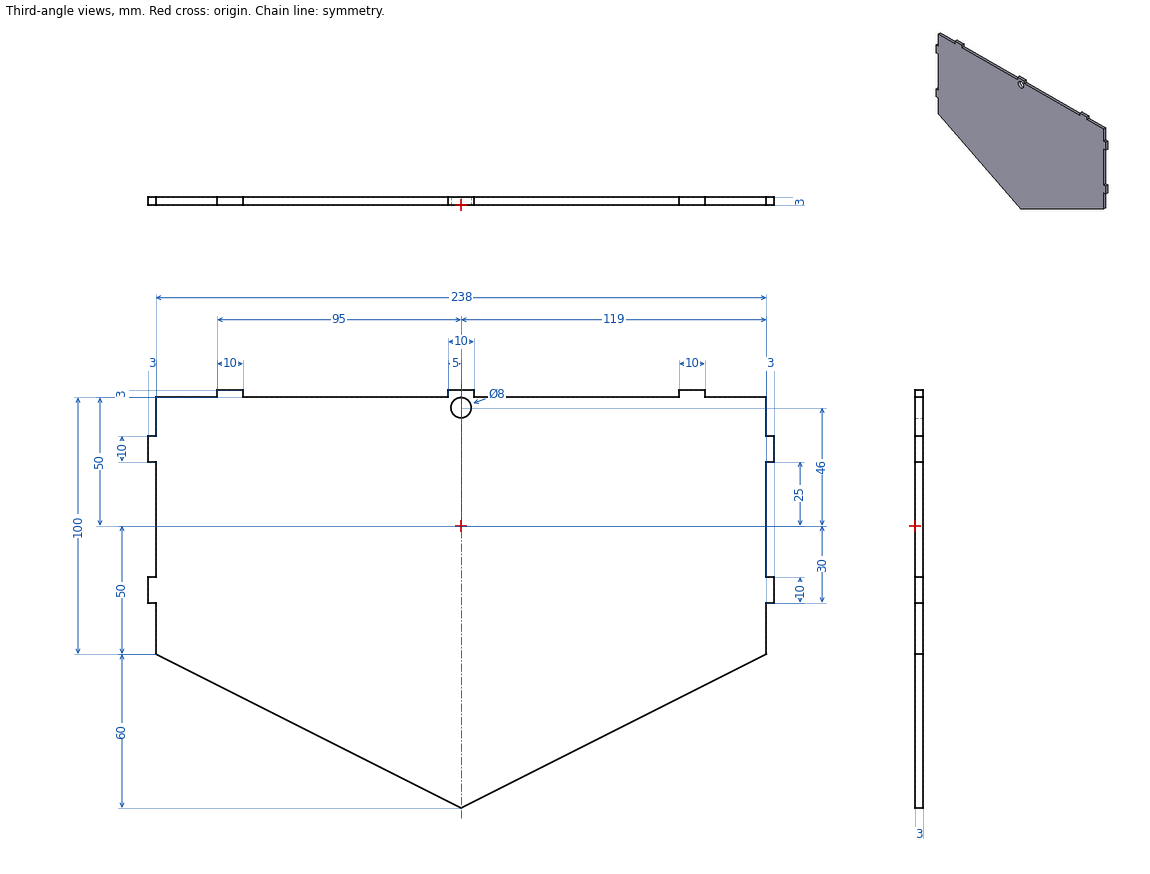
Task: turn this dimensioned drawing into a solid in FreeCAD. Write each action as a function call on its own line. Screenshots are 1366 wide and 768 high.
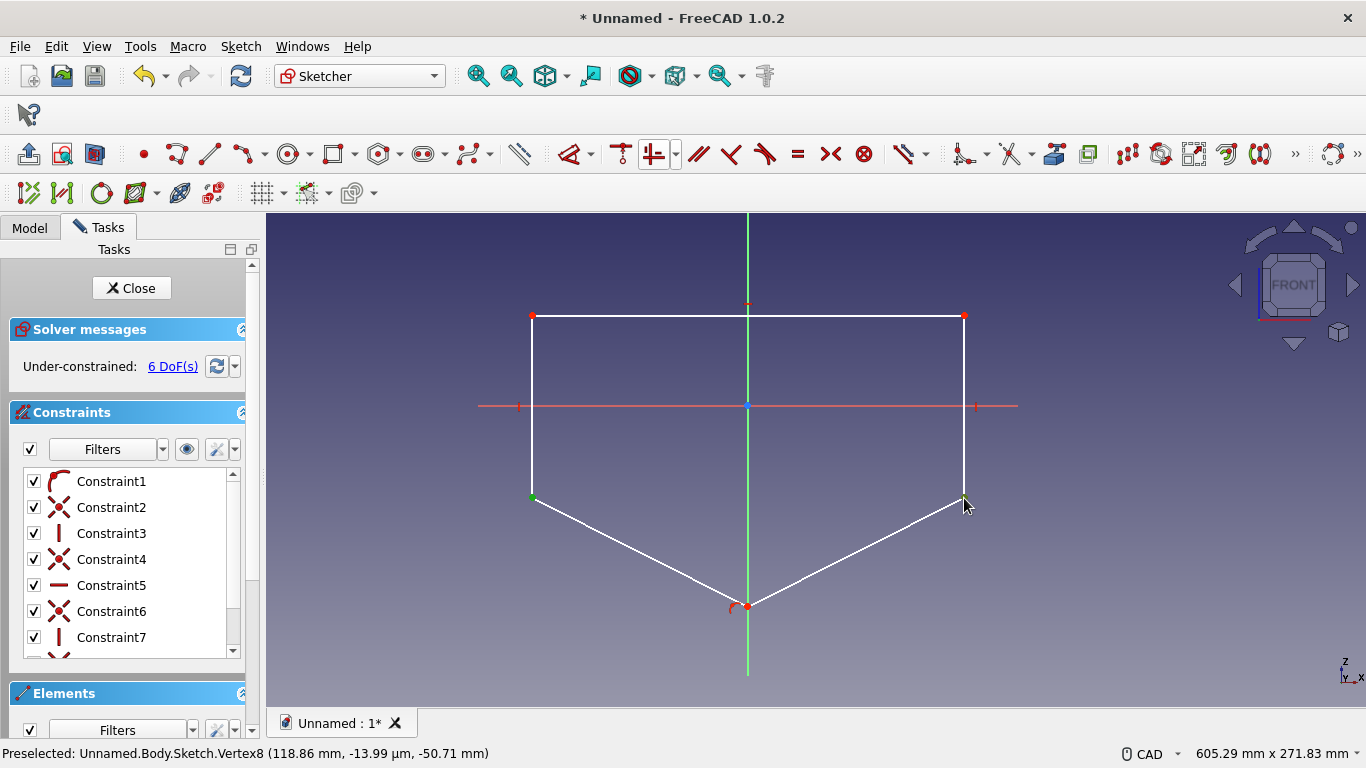
click(748, 648)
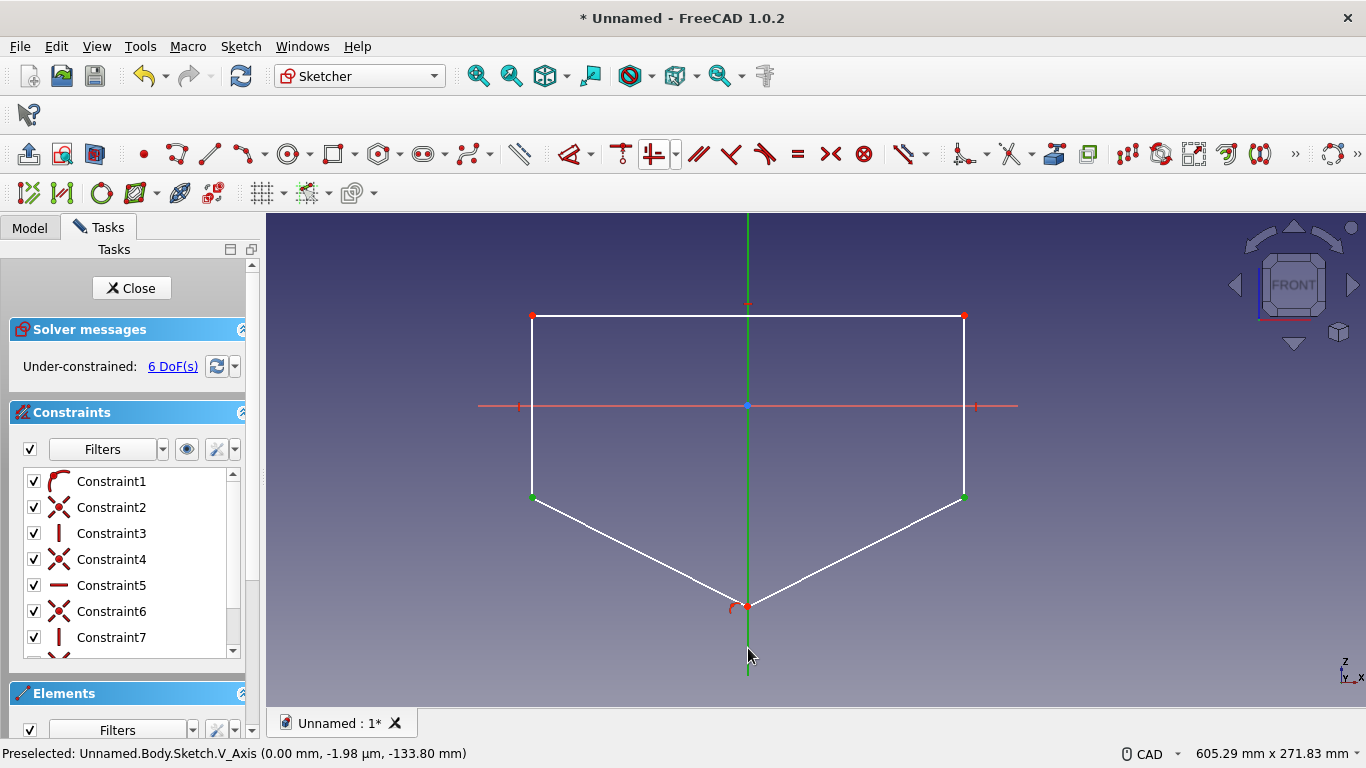
click(831, 154)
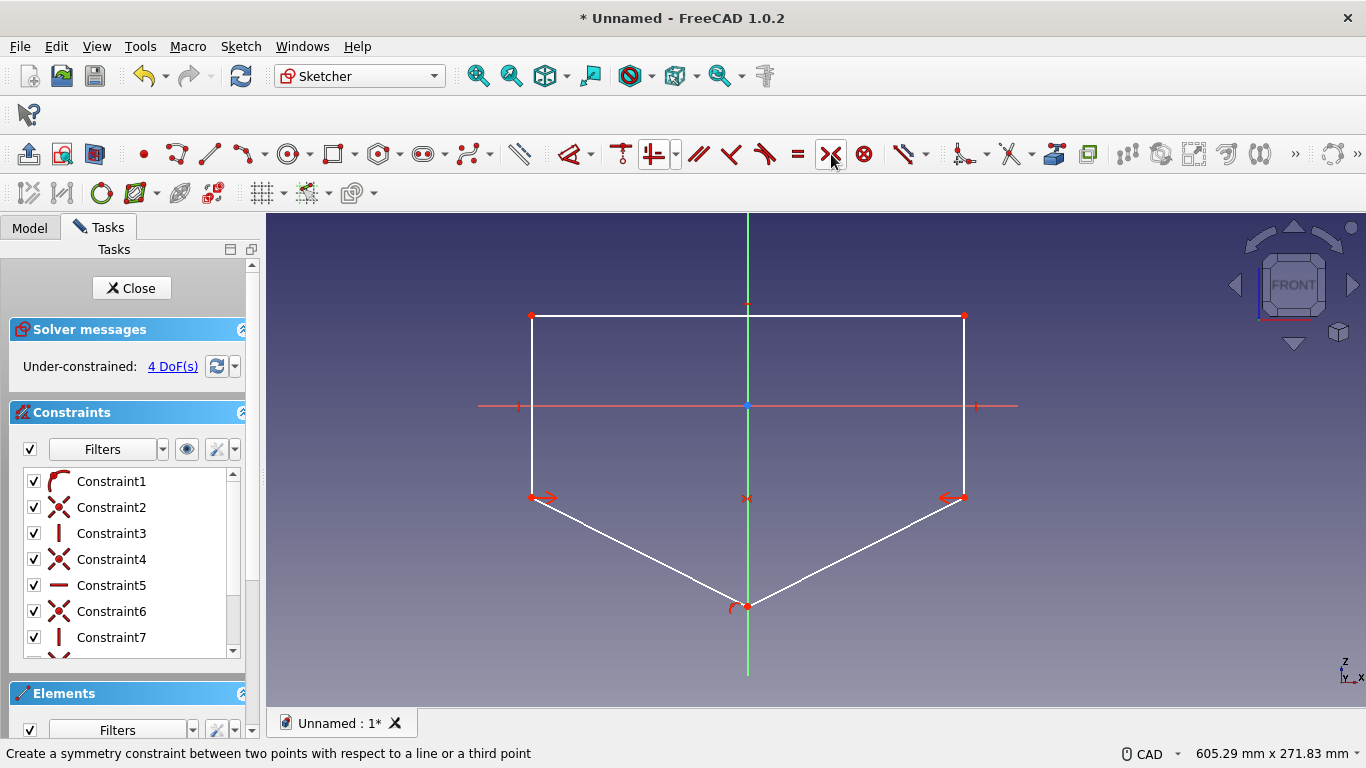
click(568, 154)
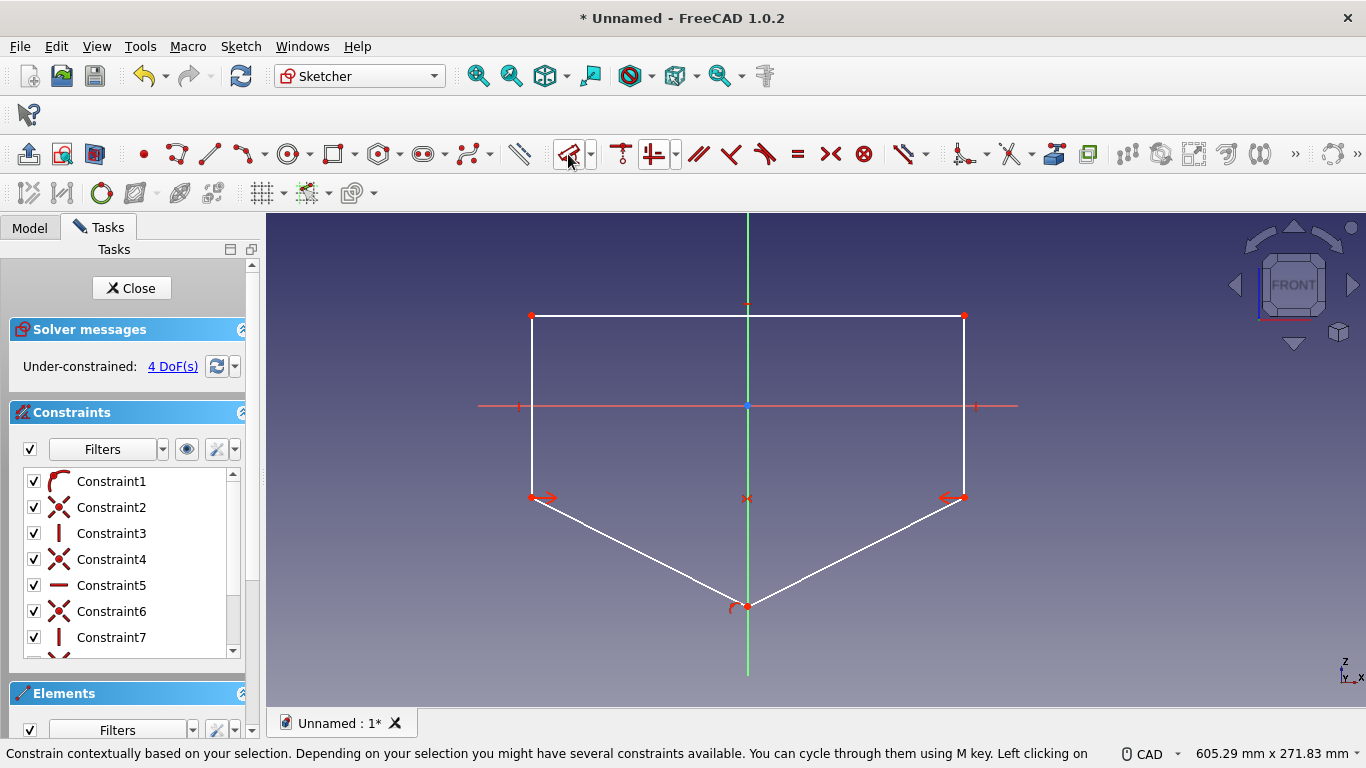
click(532, 443)
click(498, 365)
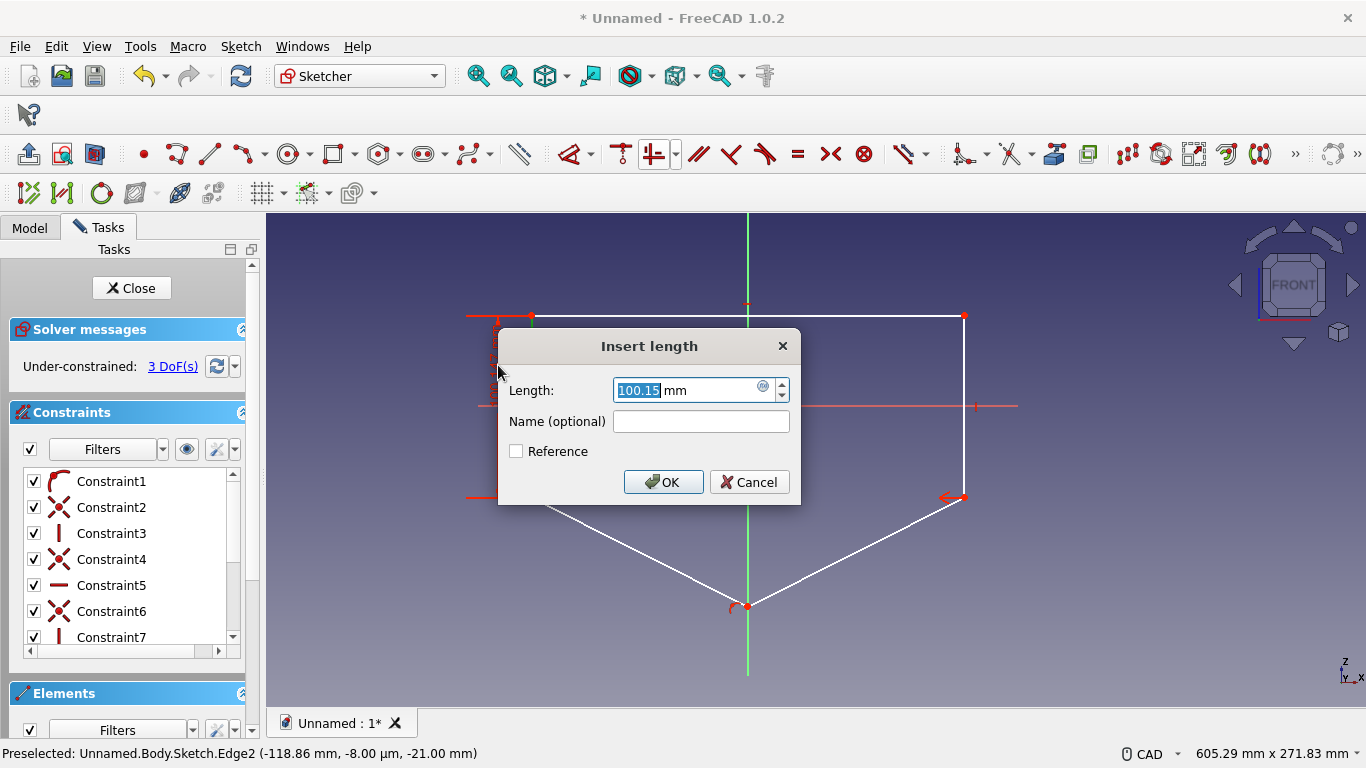
text(100)
key(Return)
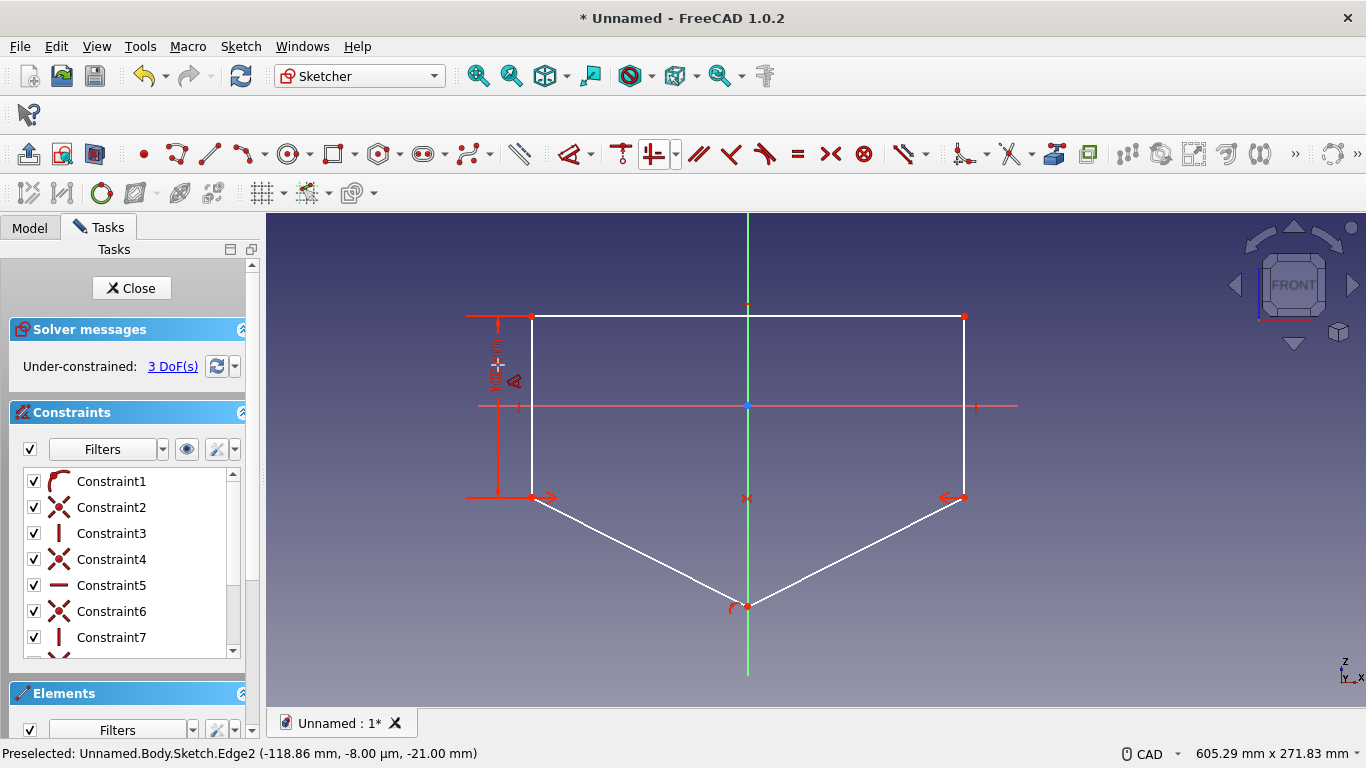
click(662, 316)
click(649, 282)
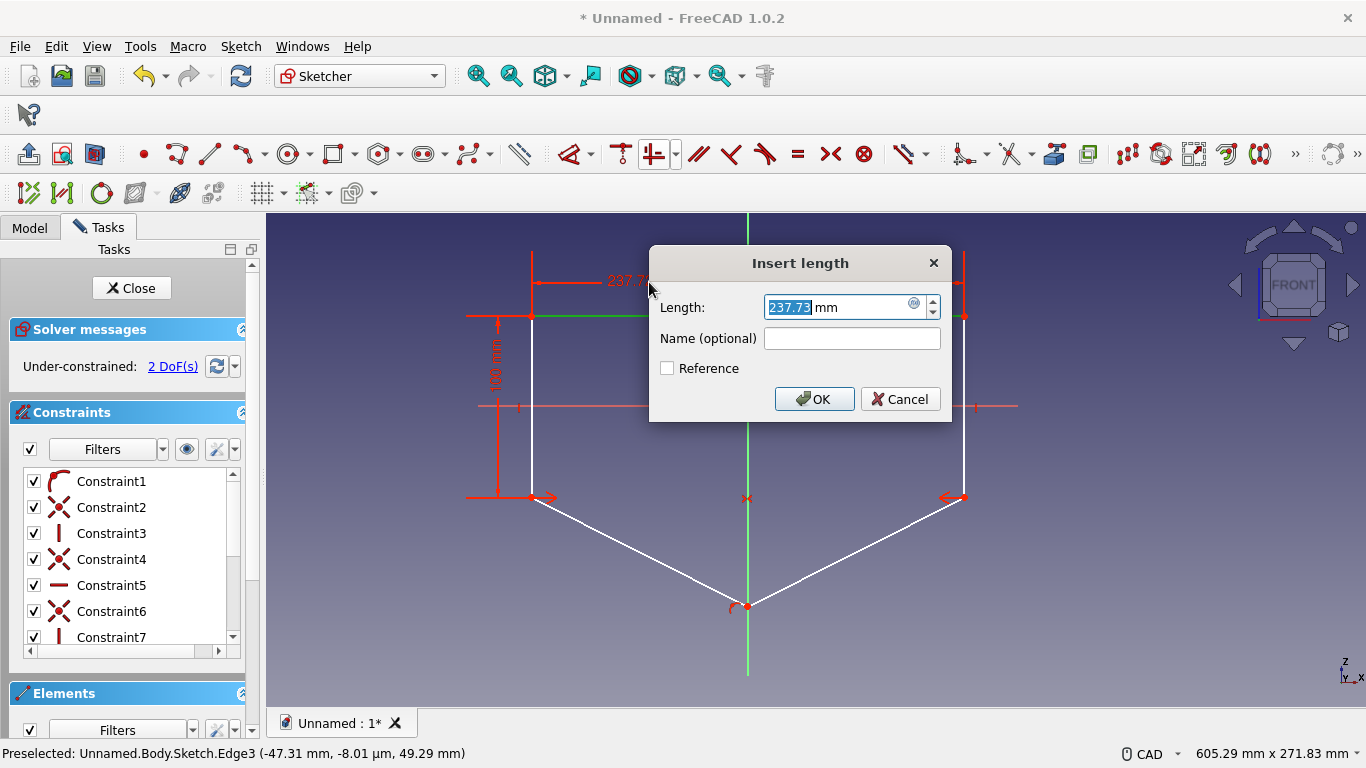
text(238)
key(Return)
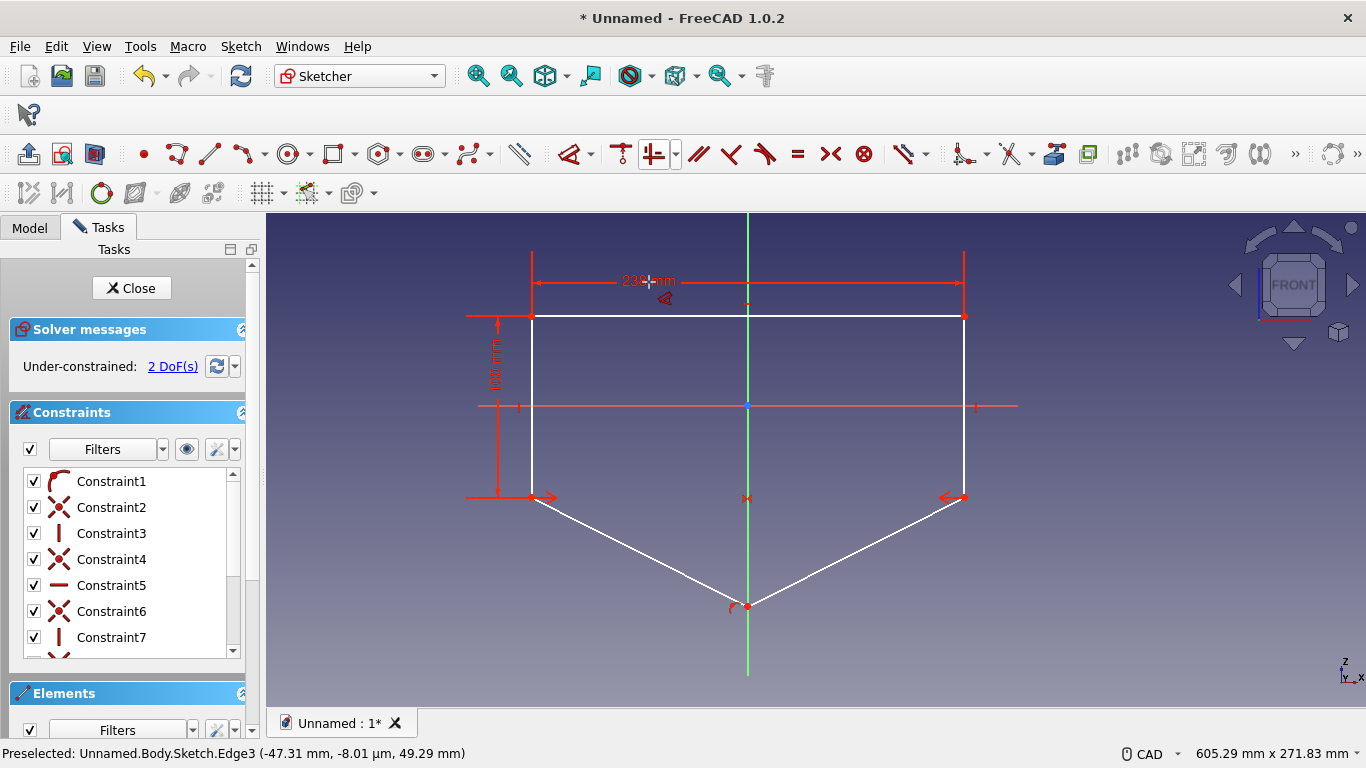
click(532, 498)
click(498, 452)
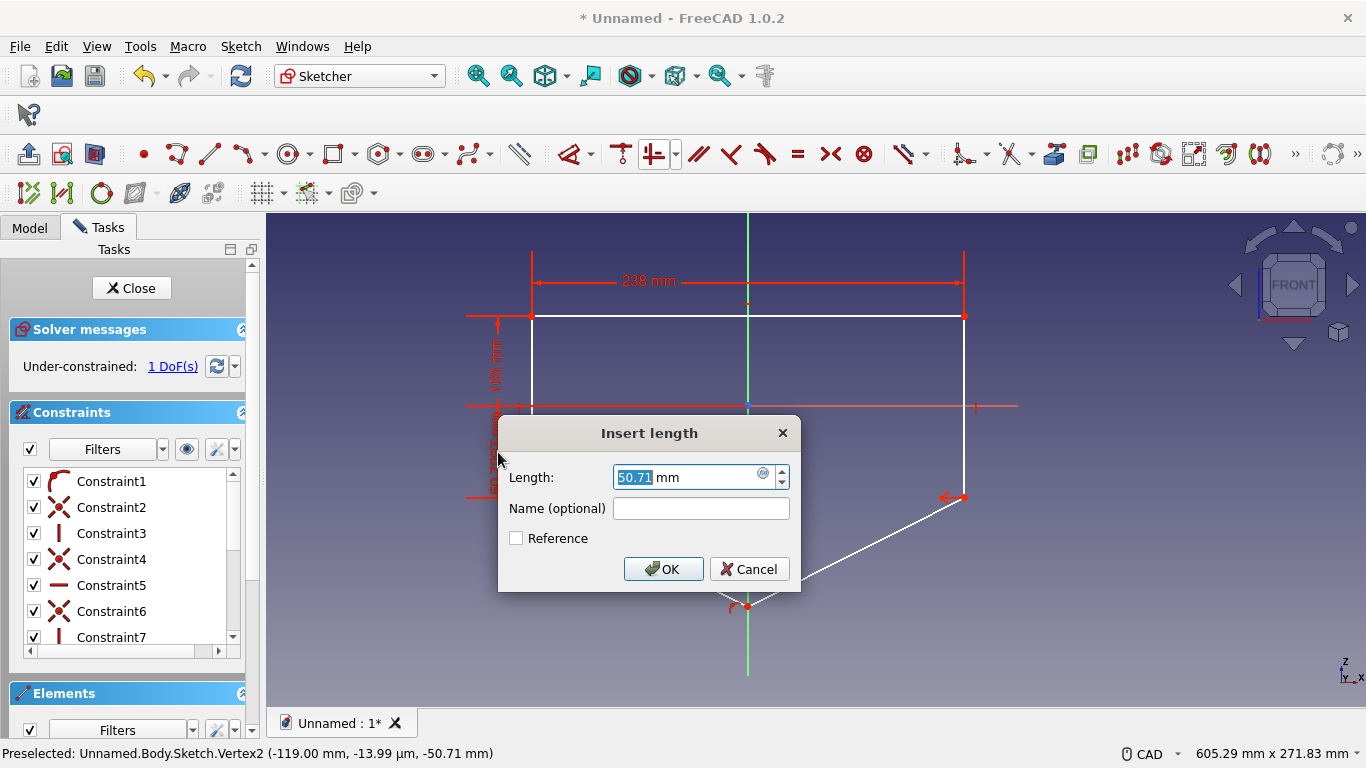
text(50)
key(Return)